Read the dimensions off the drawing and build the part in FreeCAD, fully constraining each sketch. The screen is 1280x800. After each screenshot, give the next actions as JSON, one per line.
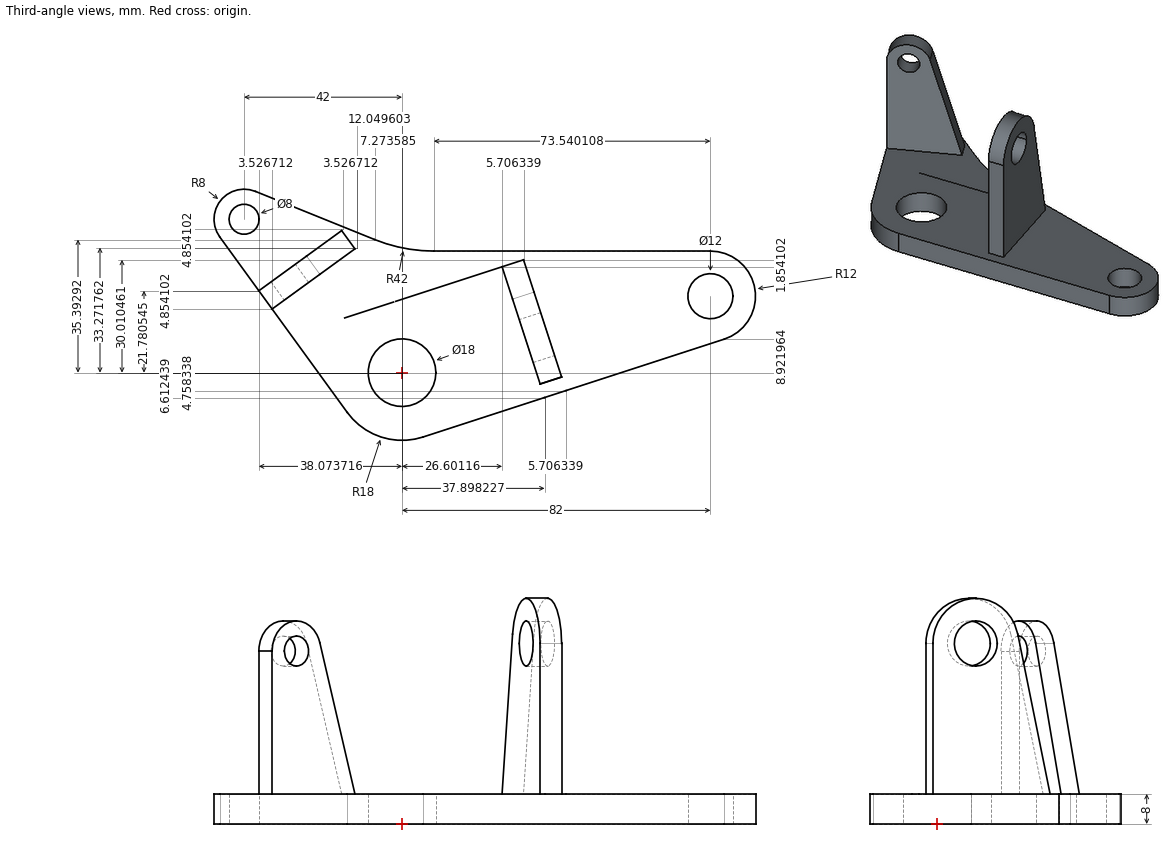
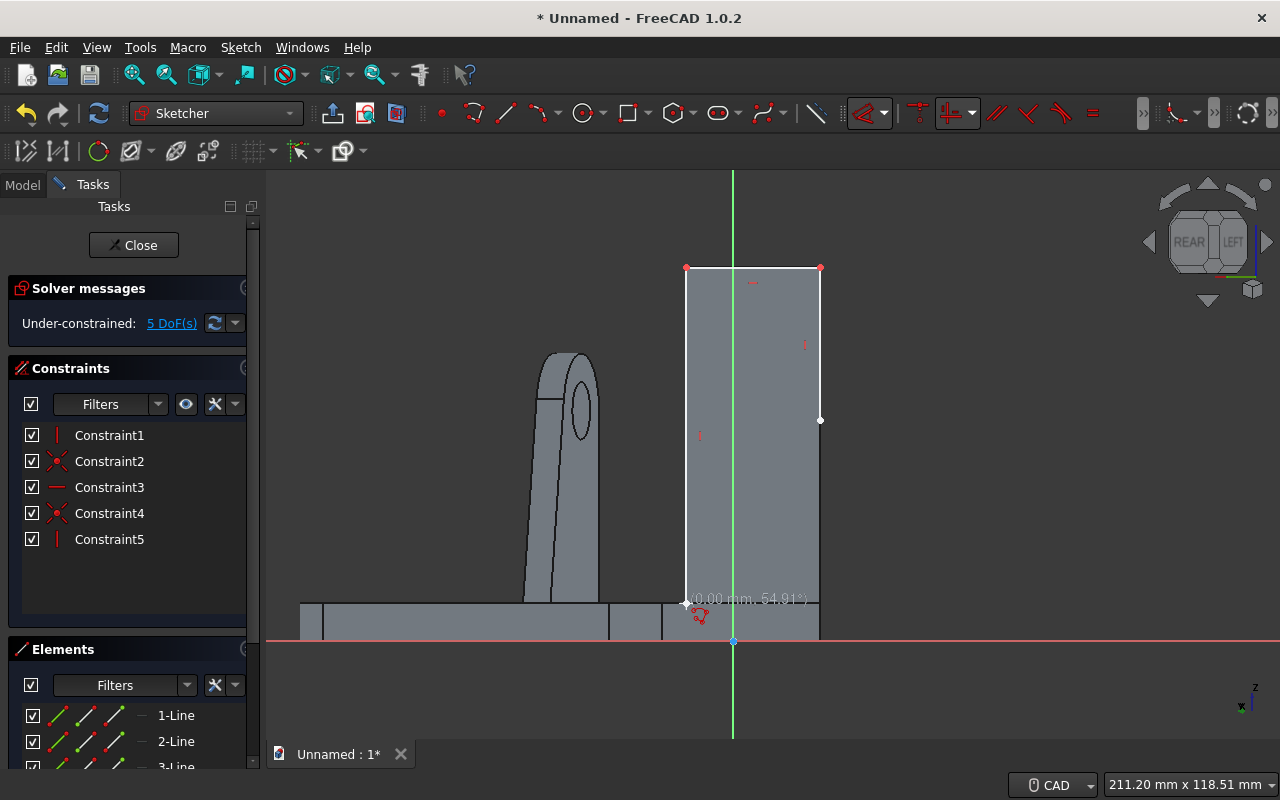
{"action": "scroll", "coordinate": [689, 603], "scroll_direction": "up", "scroll_amount": 9}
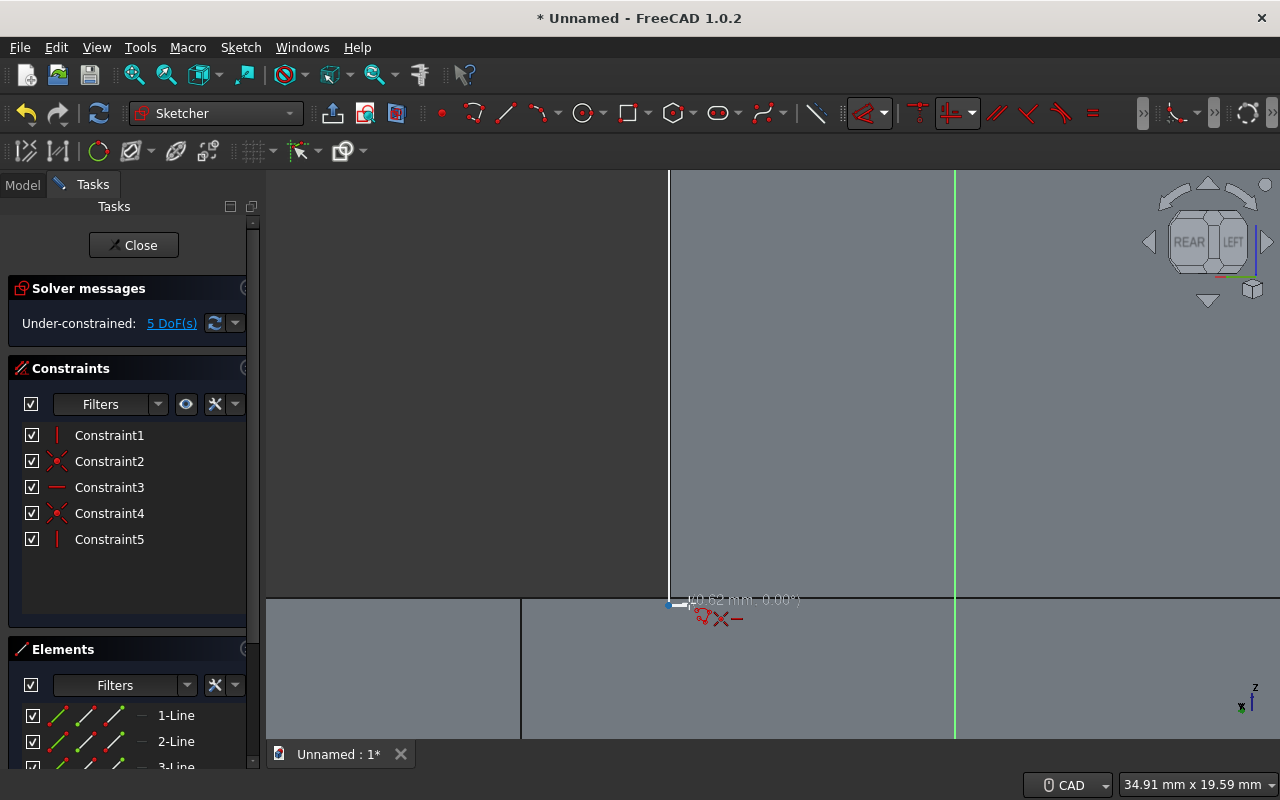
{"action": "left_click", "coordinate": [687, 599]}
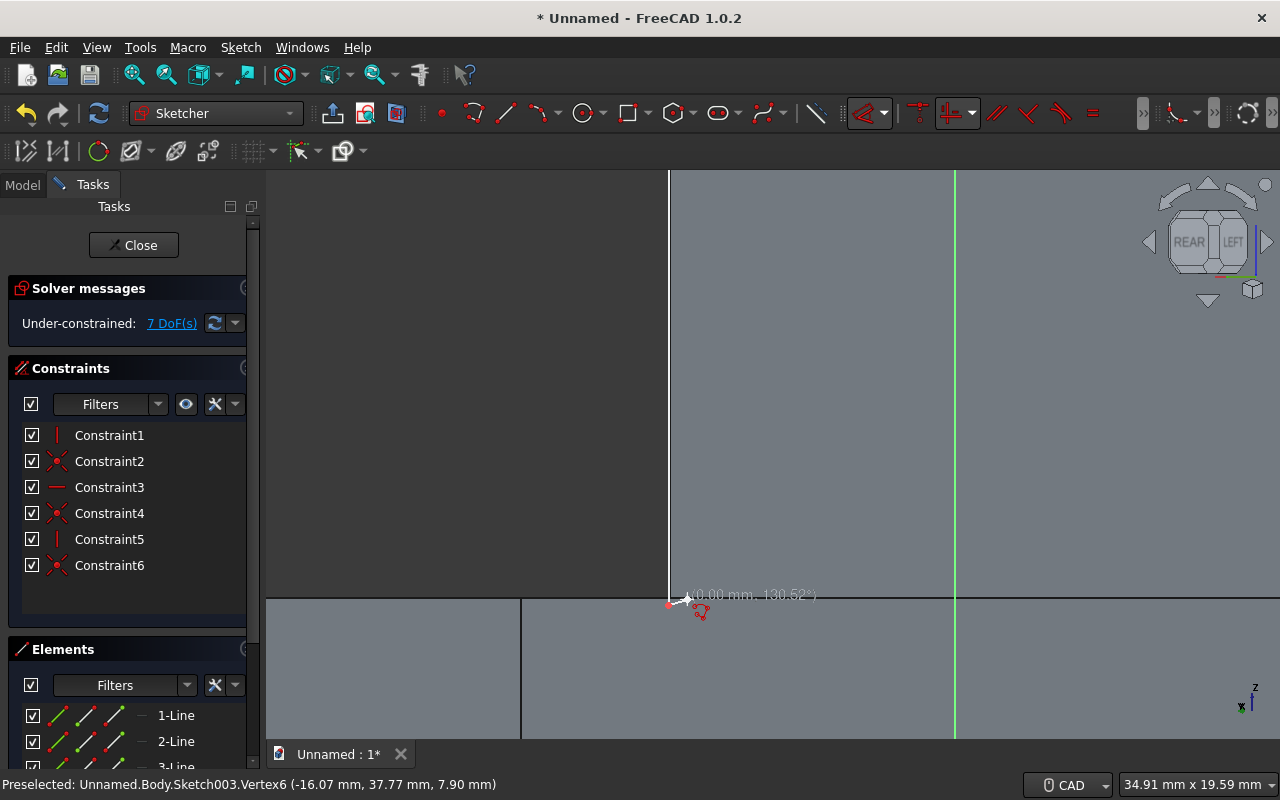
{"action": "scroll", "coordinate": [631, 604], "scroll_direction": "down", "scroll_amount": 9}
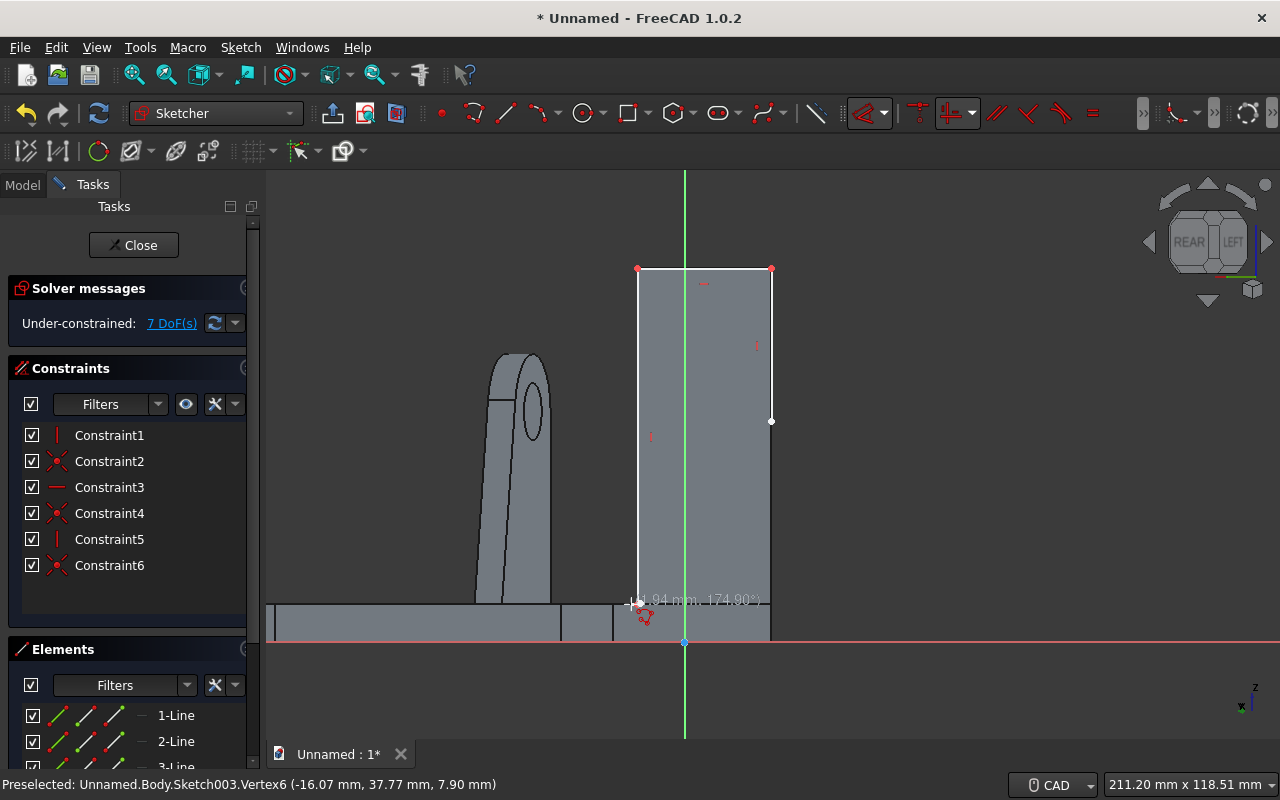
{"action": "scroll", "coordinate": [696, 411], "scroll_direction": "up", "scroll_amount": 2}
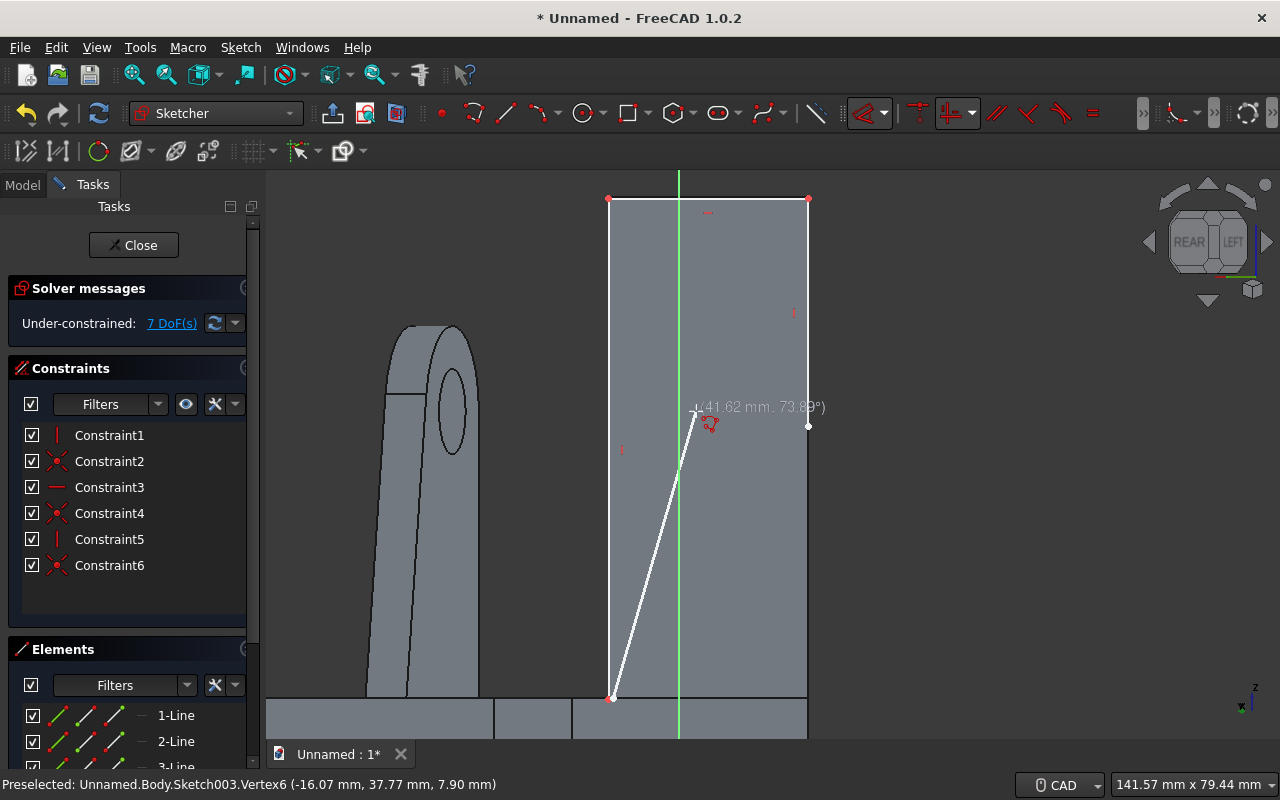
{"action": "left_click", "coordinate": [696, 410]}
{"action": "right_click", "coordinate": [696, 410]}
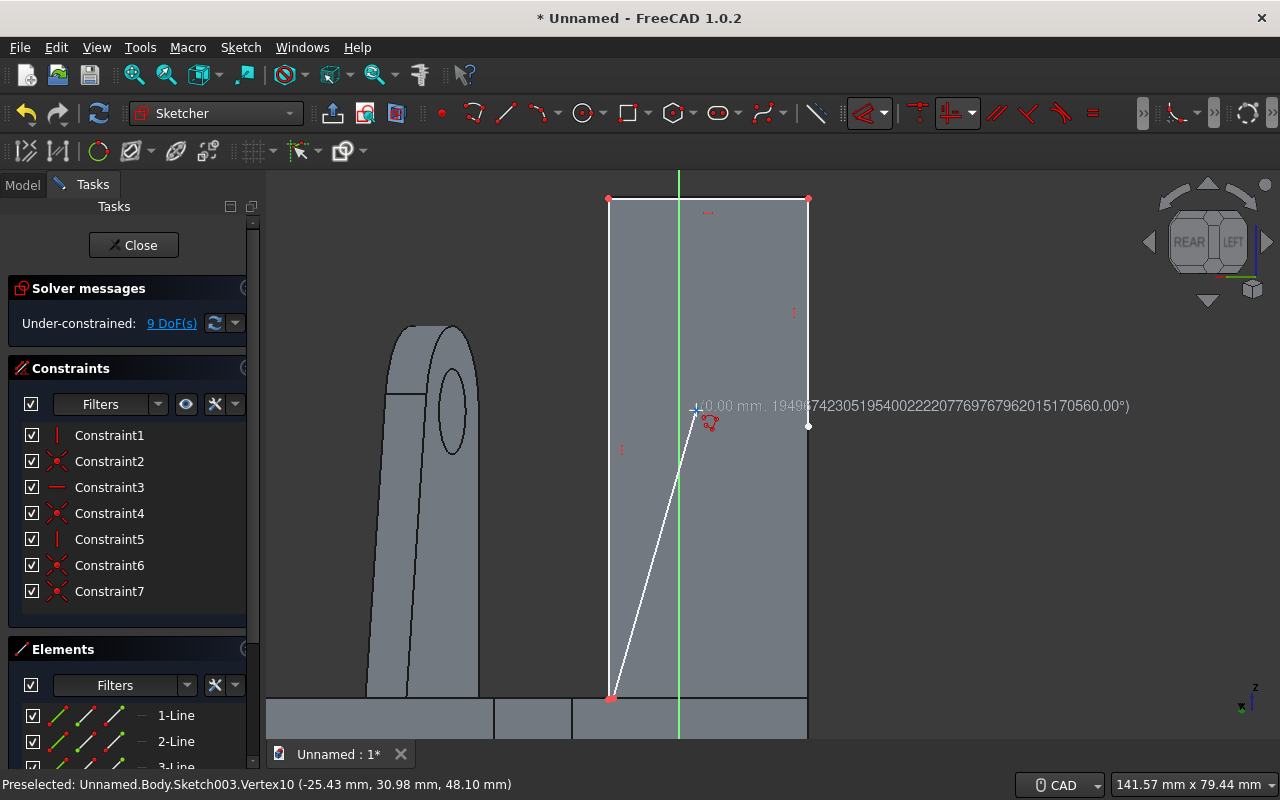
{"action": "left_click", "coordinate": [538, 114]}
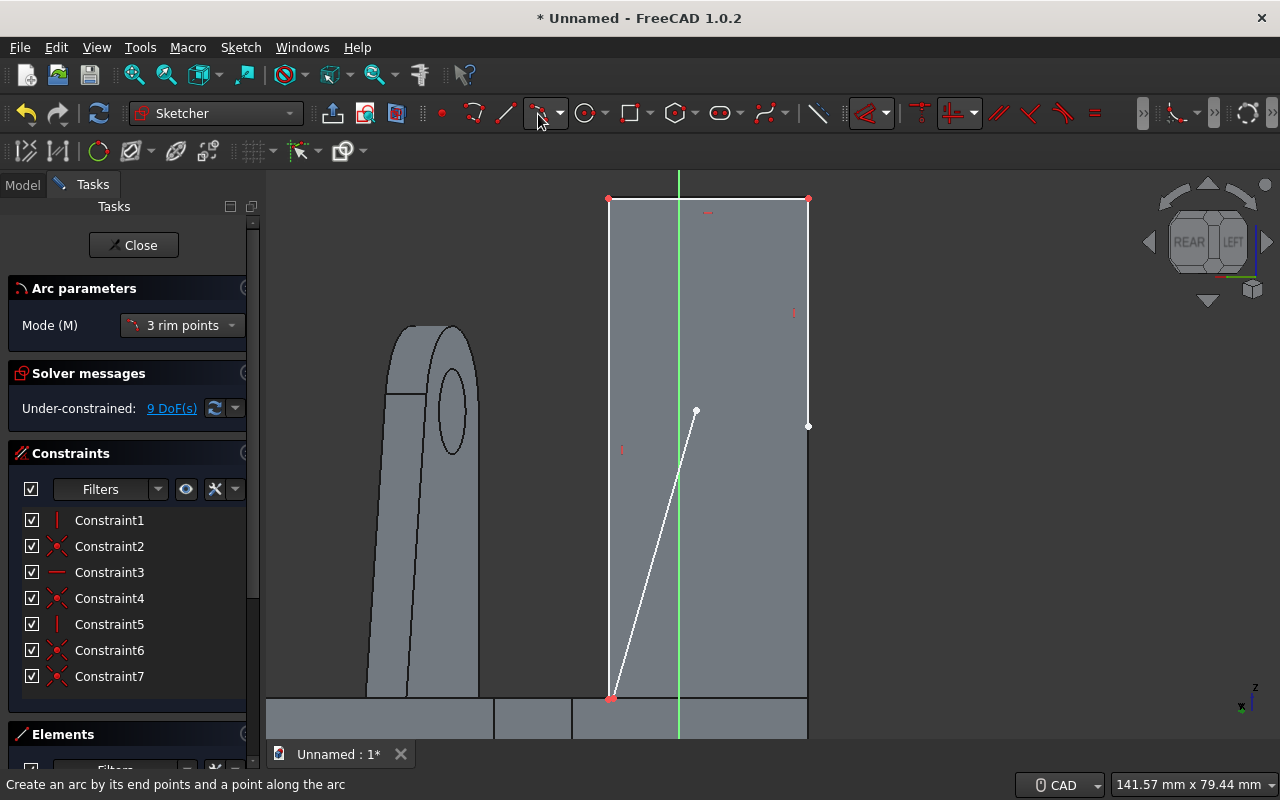
{"action": "left_click", "coordinate": [696, 411]}
{"action": "left_click", "coordinate": [808, 427]}
{"action": "left_click", "coordinate": [759, 369]}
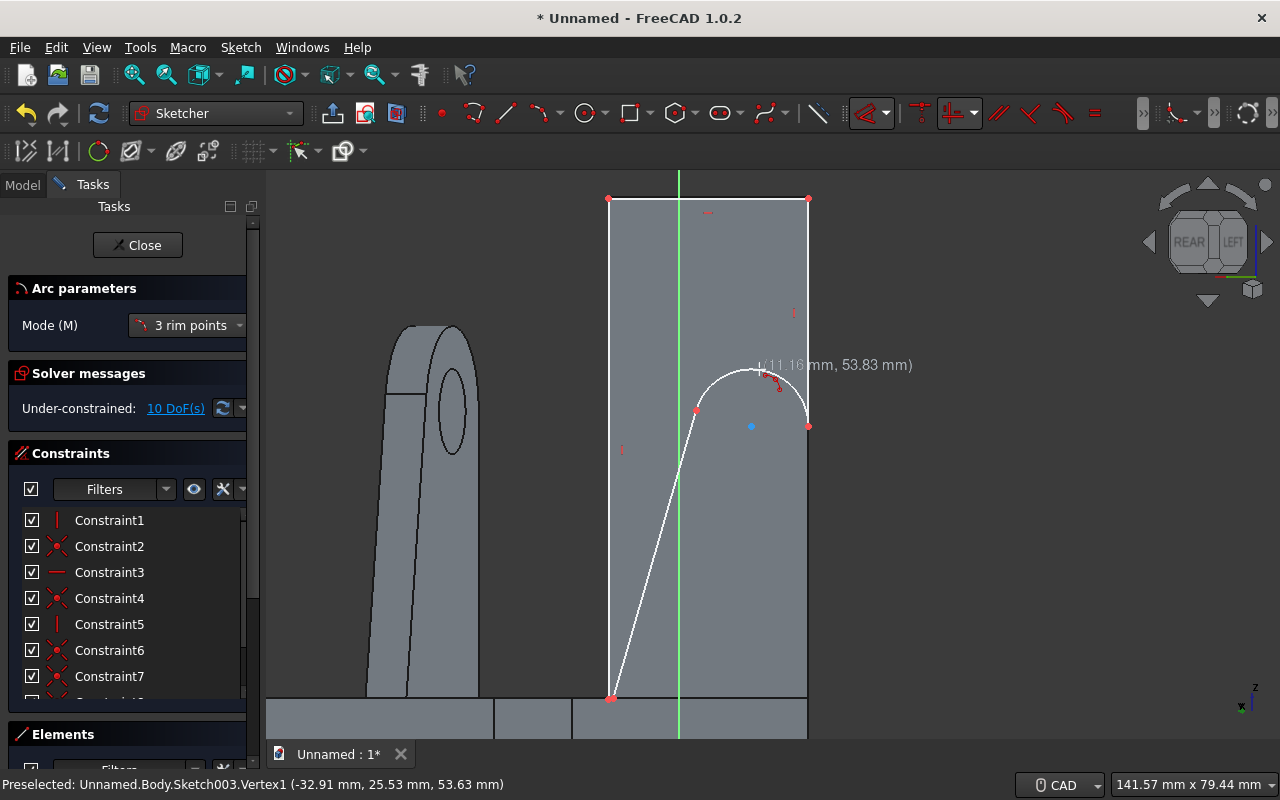
{"action": "key", "text": "g c"}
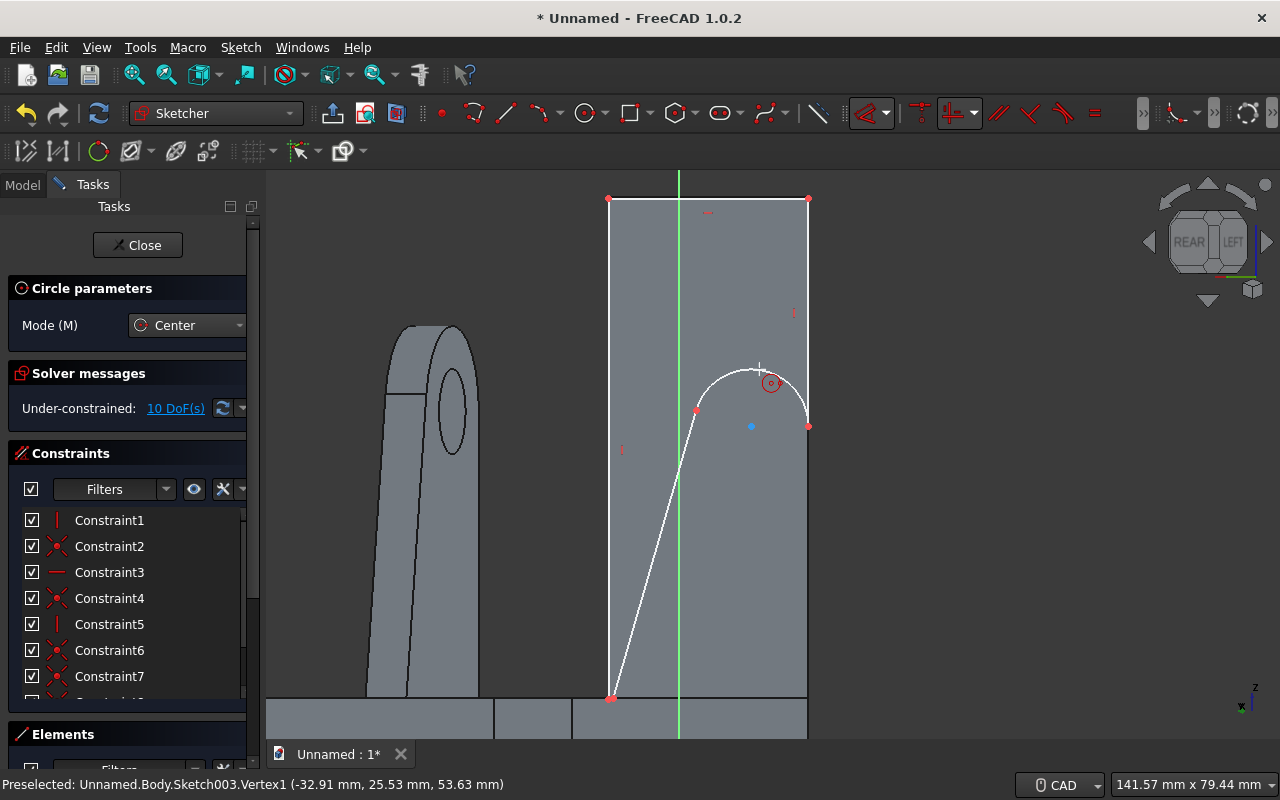
{"action": "left_click", "coordinate": [751, 426]}
{"action": "left_click", "coordinate": [771, 406]}
{"action": "key", "text": "Escape"}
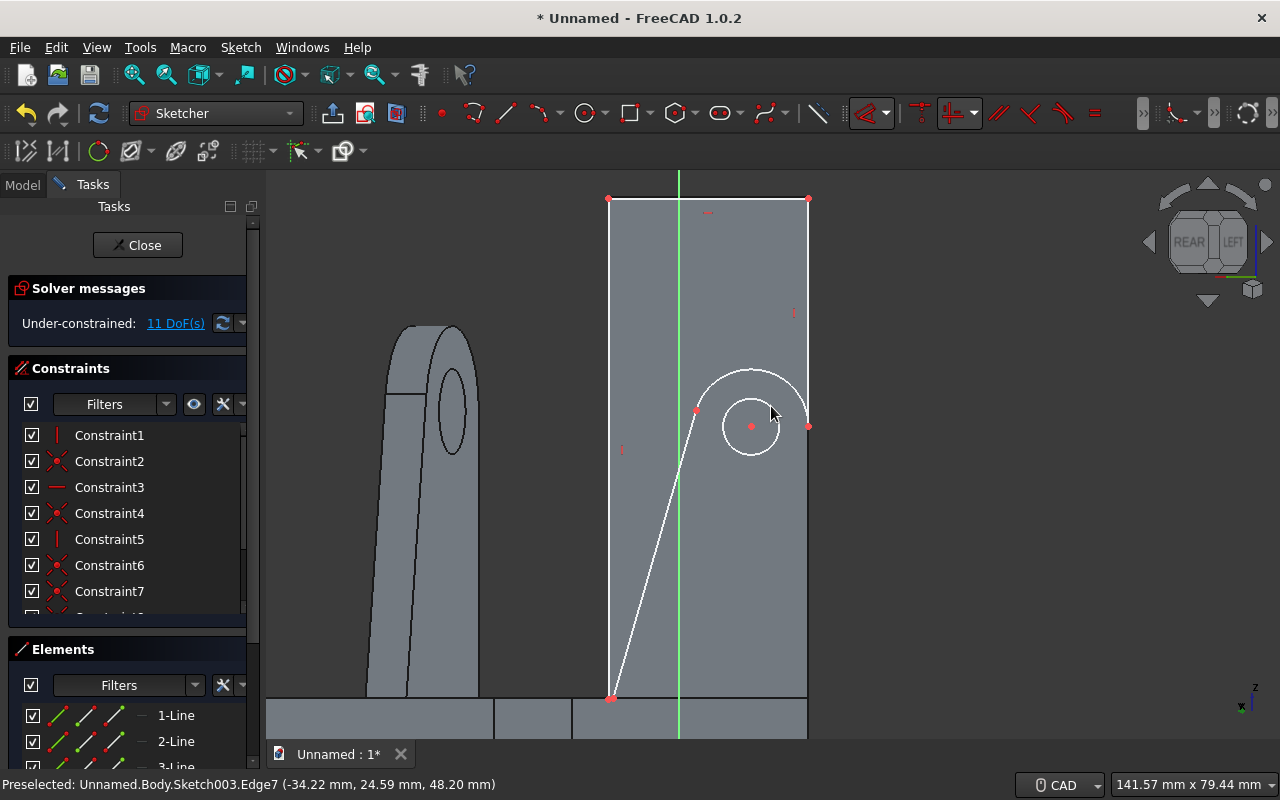
{"action": "left_click", "coordinate": [808, 358]}